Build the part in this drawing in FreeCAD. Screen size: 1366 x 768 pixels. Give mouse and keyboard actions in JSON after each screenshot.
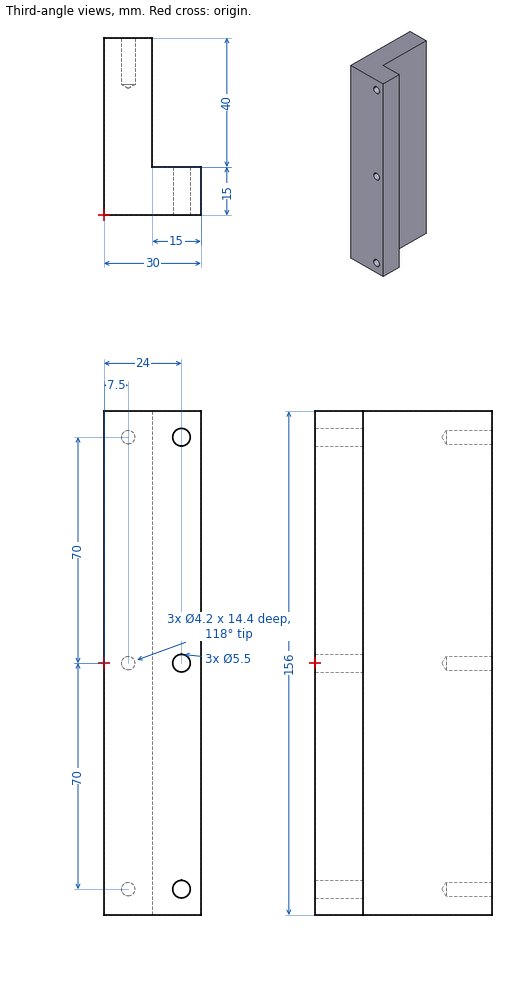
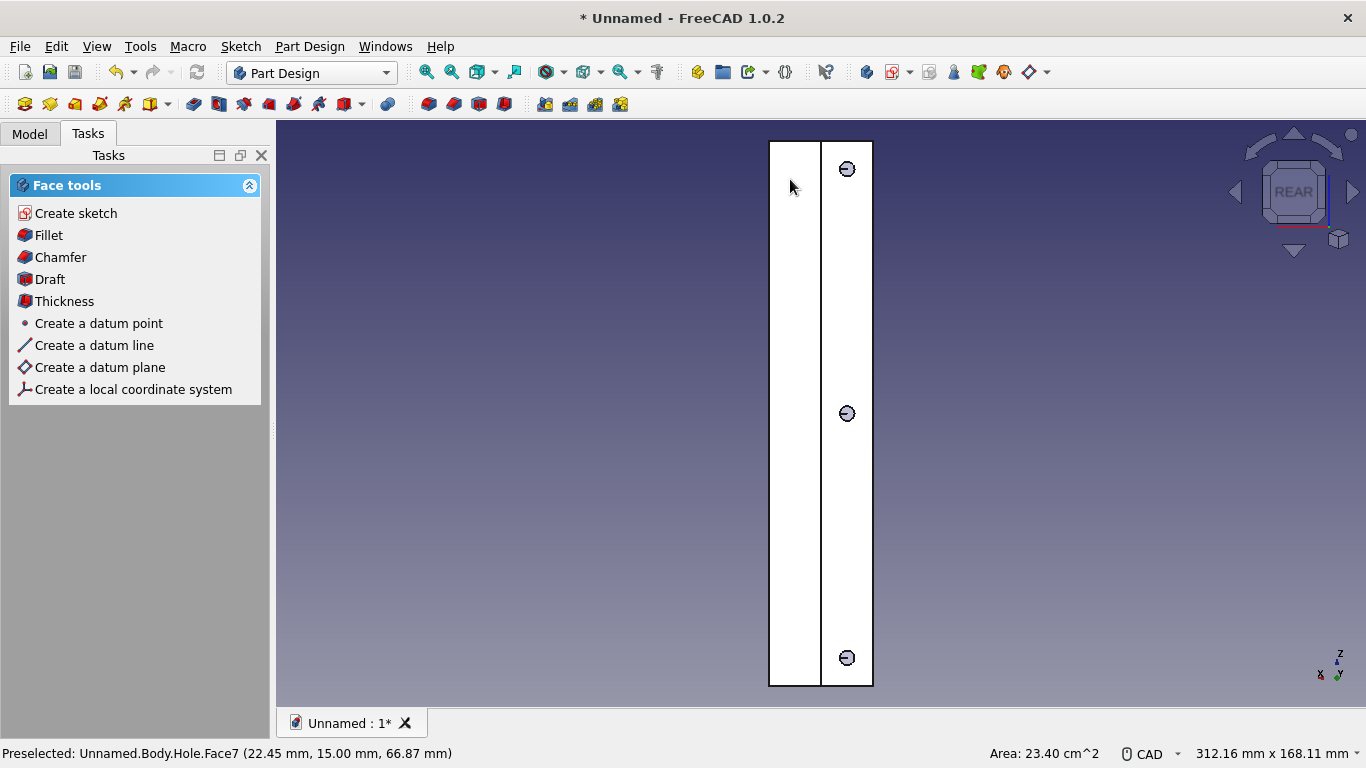
{"action": "left_click", "coordinate": [892, 72]}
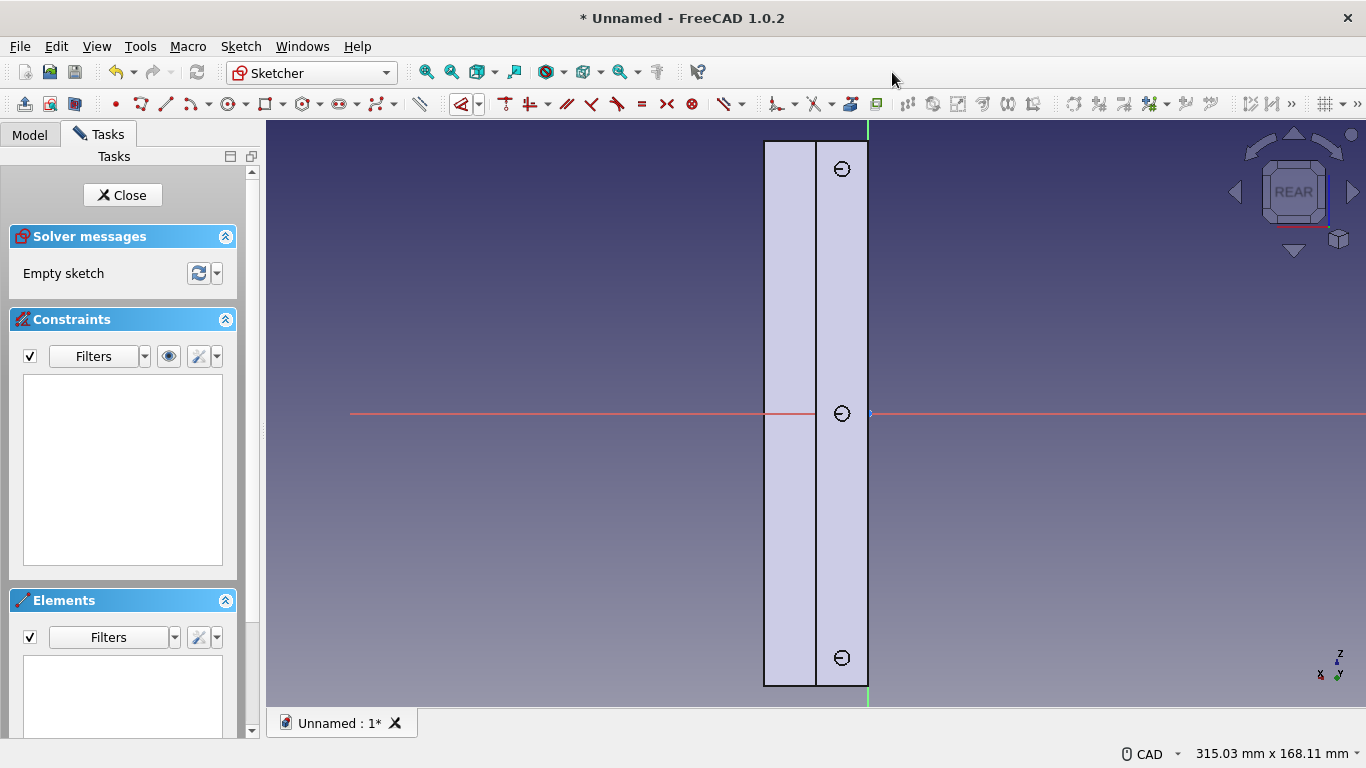
{"action": "left_click", "coordinate": [75, 104]}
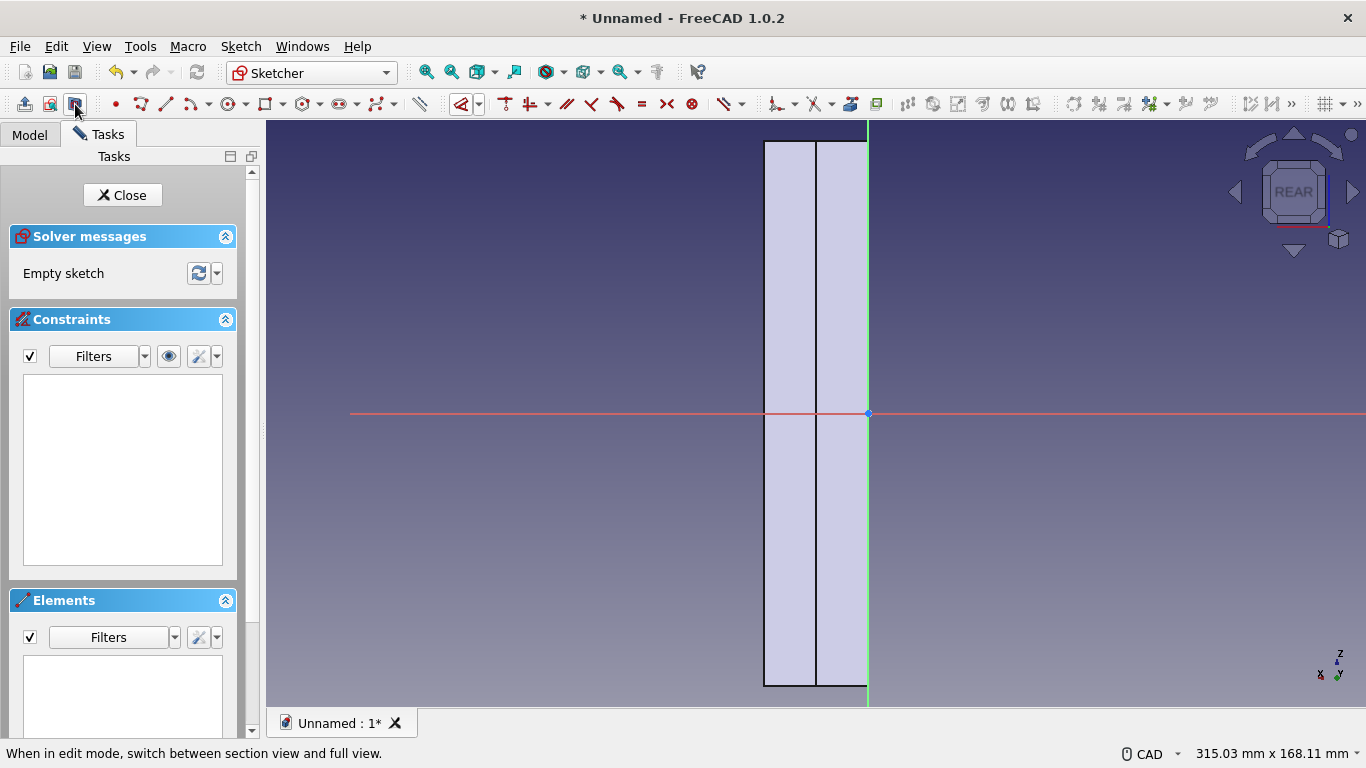
{"action": "scroll", "coordinate": [597, 413], "scroll_direction": "down", "scroll_amount": 2}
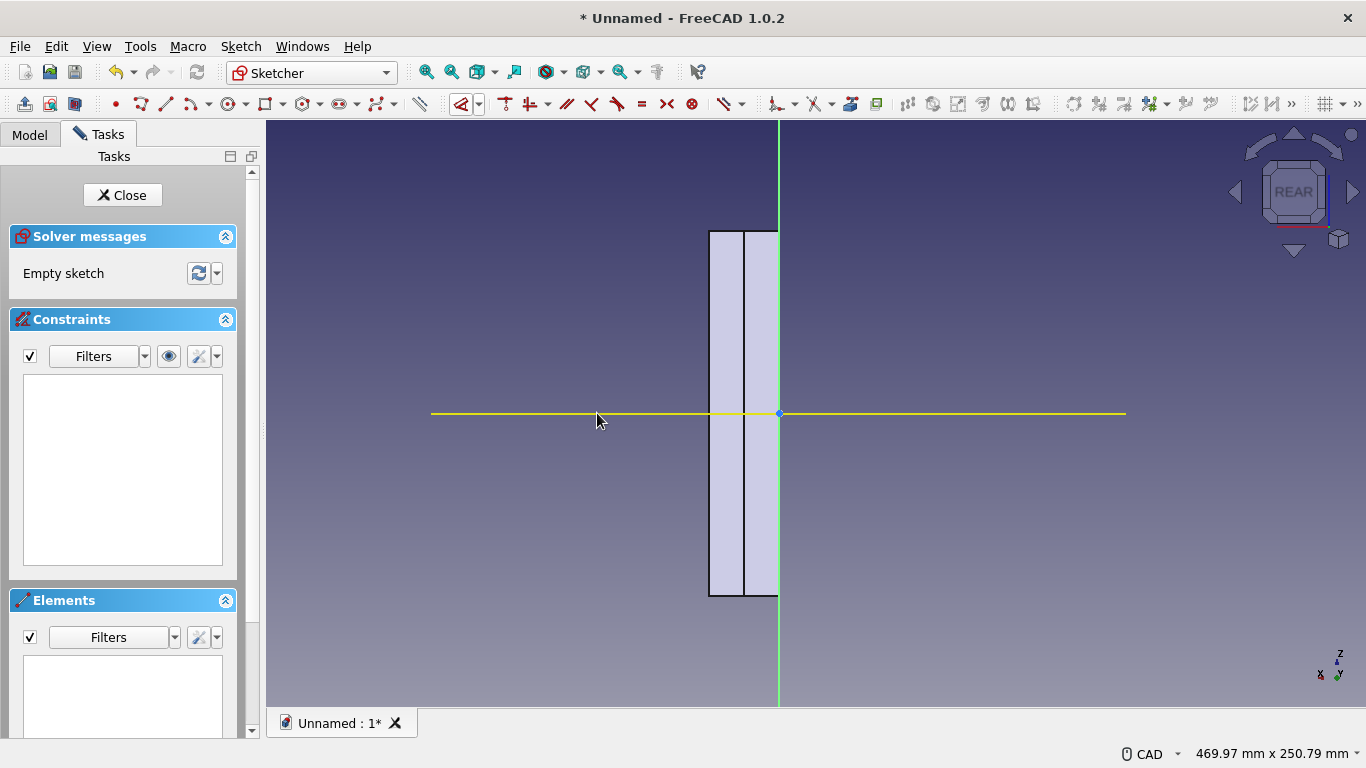
{"action": "left_click", "coordinate": [228, 104]}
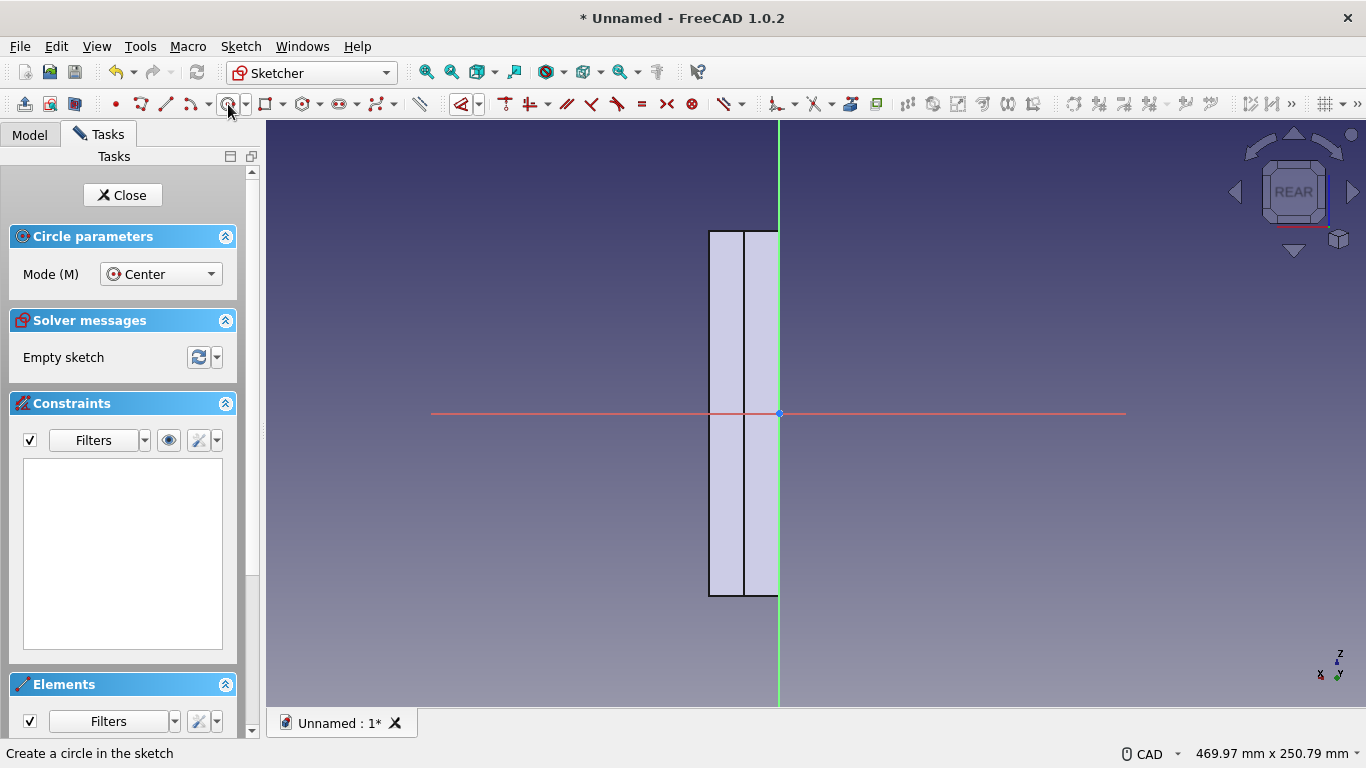
{"action": "scroll", "coordinate": [723, 414], "scroll_direction": "up", "scroll_amount": 7}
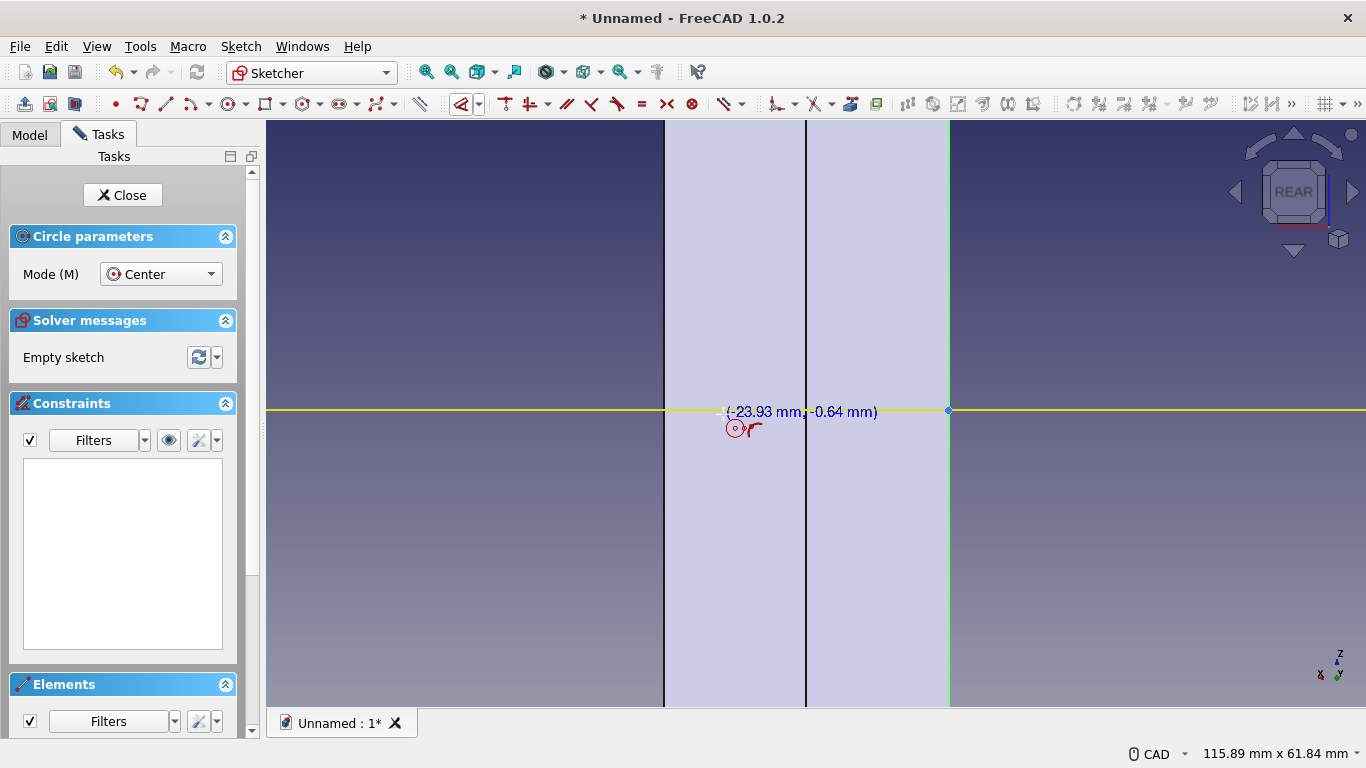
{"action": "scroll", "coordinate": [723, 415], "scroll_direction": "down", "scroll_amount": 7}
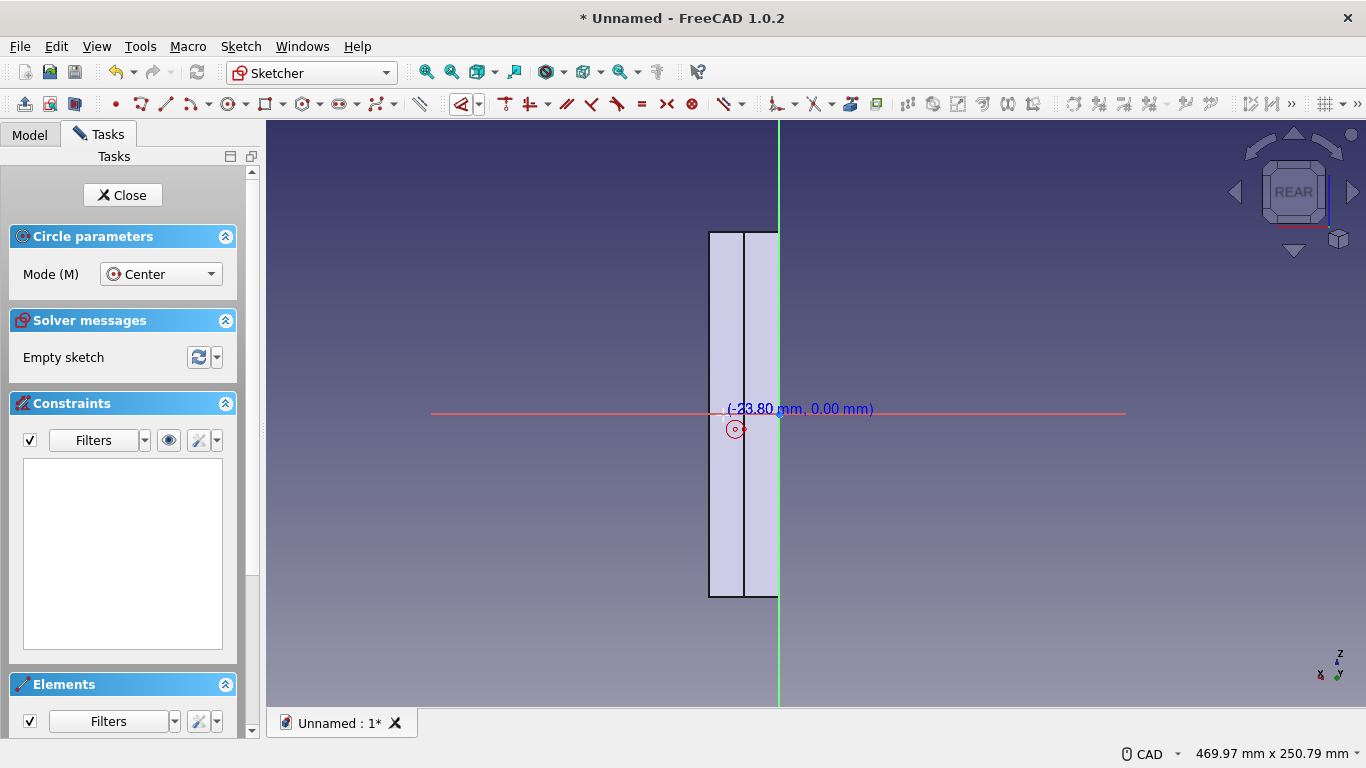
{"action": "left_click", "coordinate": [723, 414]}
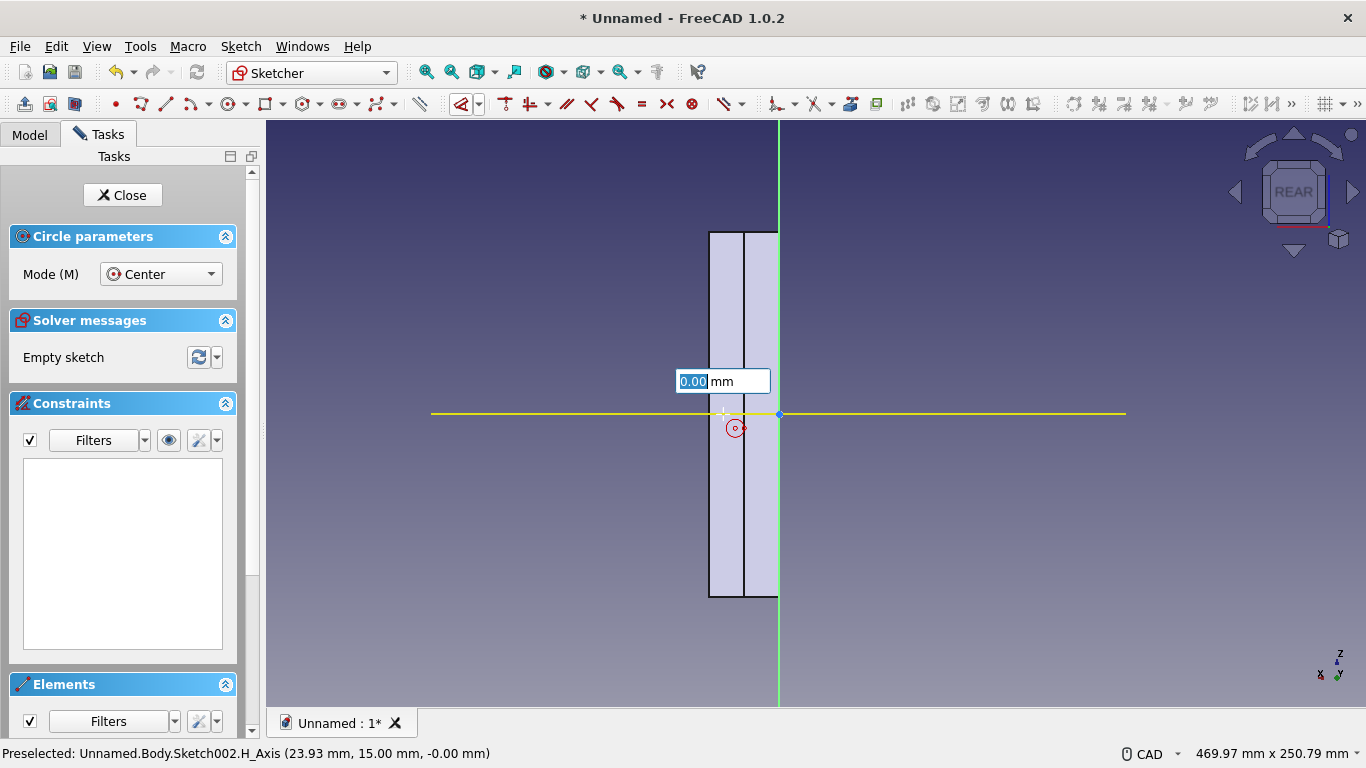
{"action": "scroll", "coordinate": [725, 408], "scroll_direction": "up", "scroll_amount": 5}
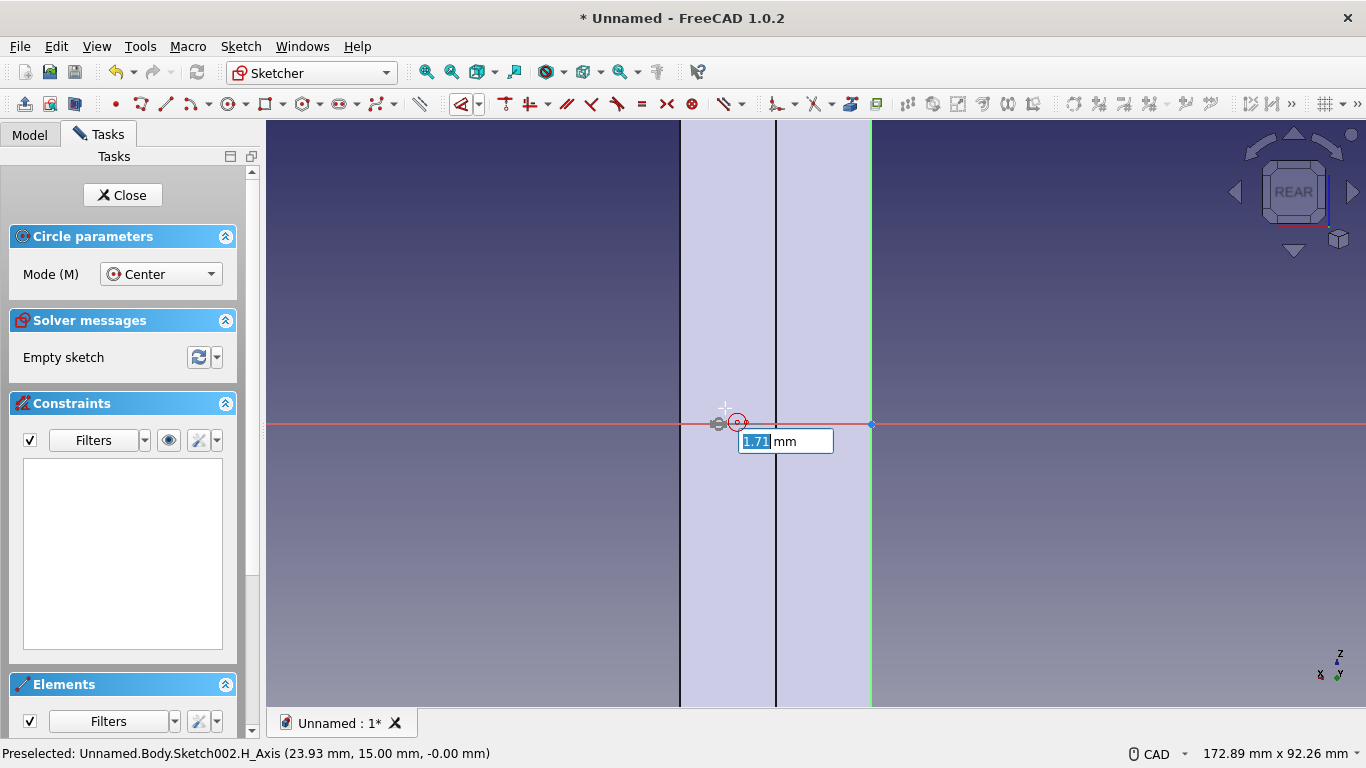
{"action": "left_click", "coordinate": [724, 408]}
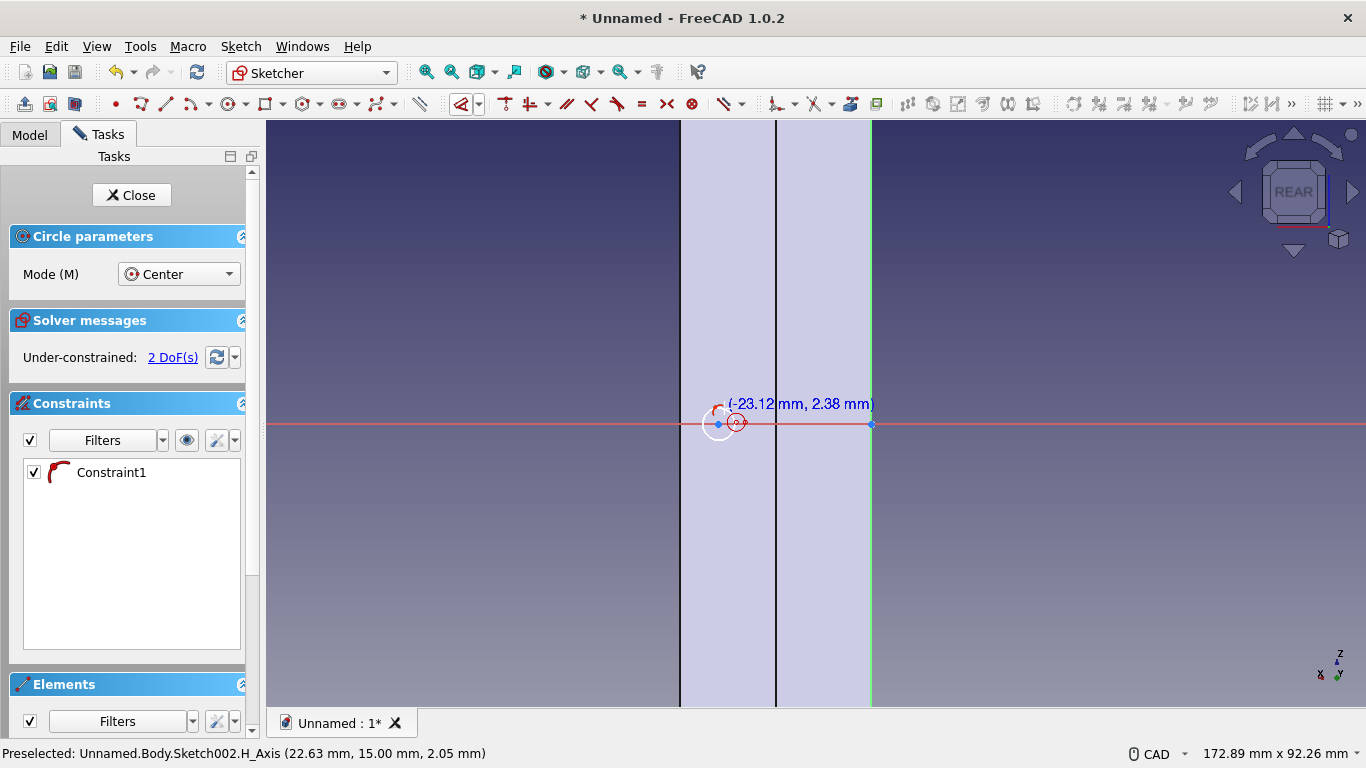
{"action": "scroll", "coordinate": [725, 407], "scroll_direction": "down", "scroll_amount": 5}